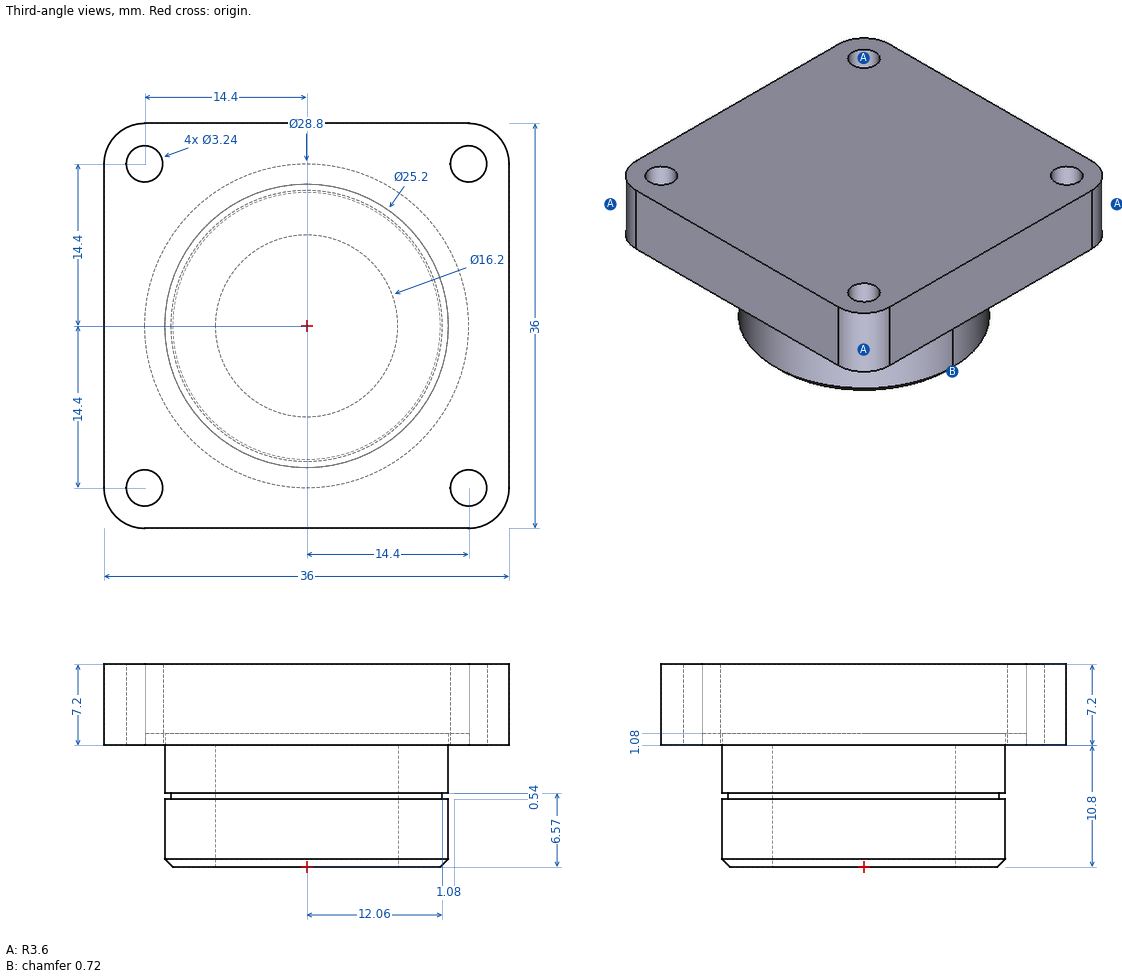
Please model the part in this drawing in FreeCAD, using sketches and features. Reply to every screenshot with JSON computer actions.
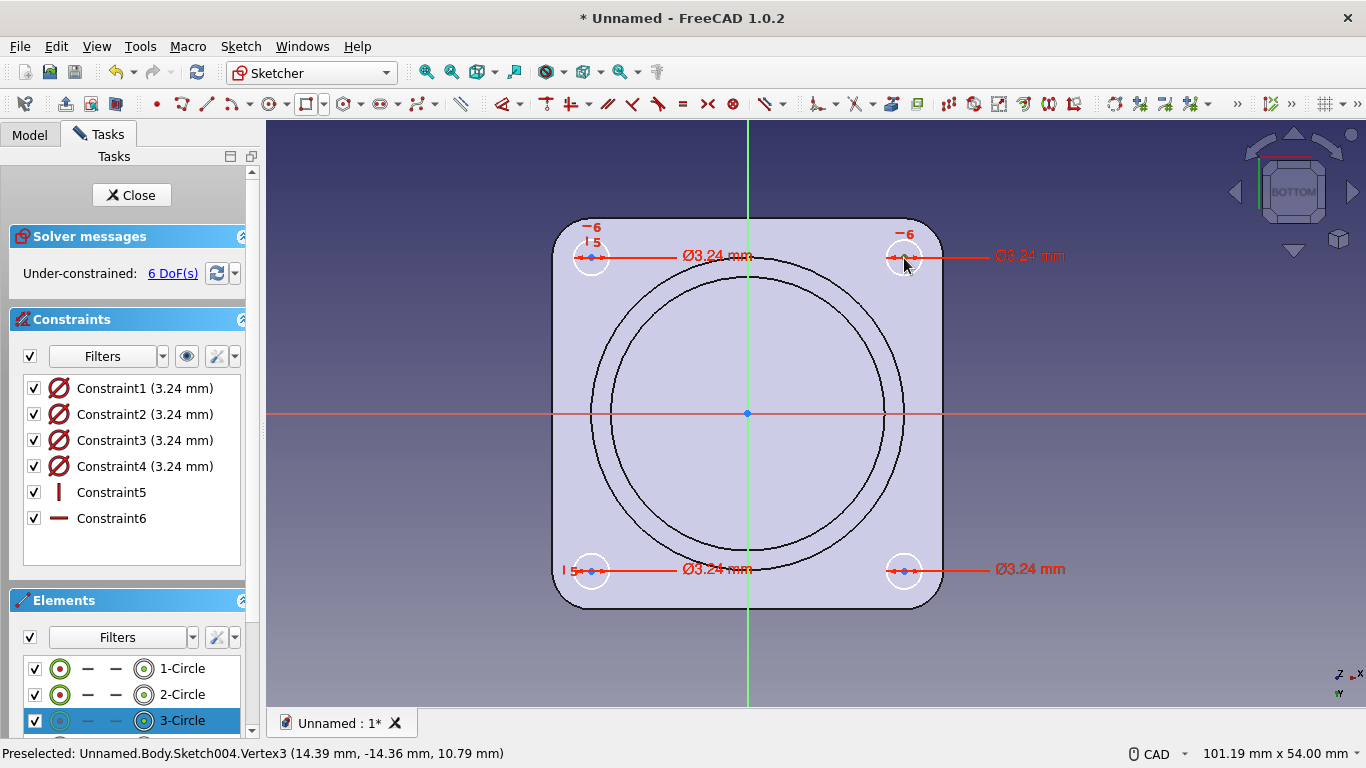
{"action": "left_click", "coordinate": [904, 571]}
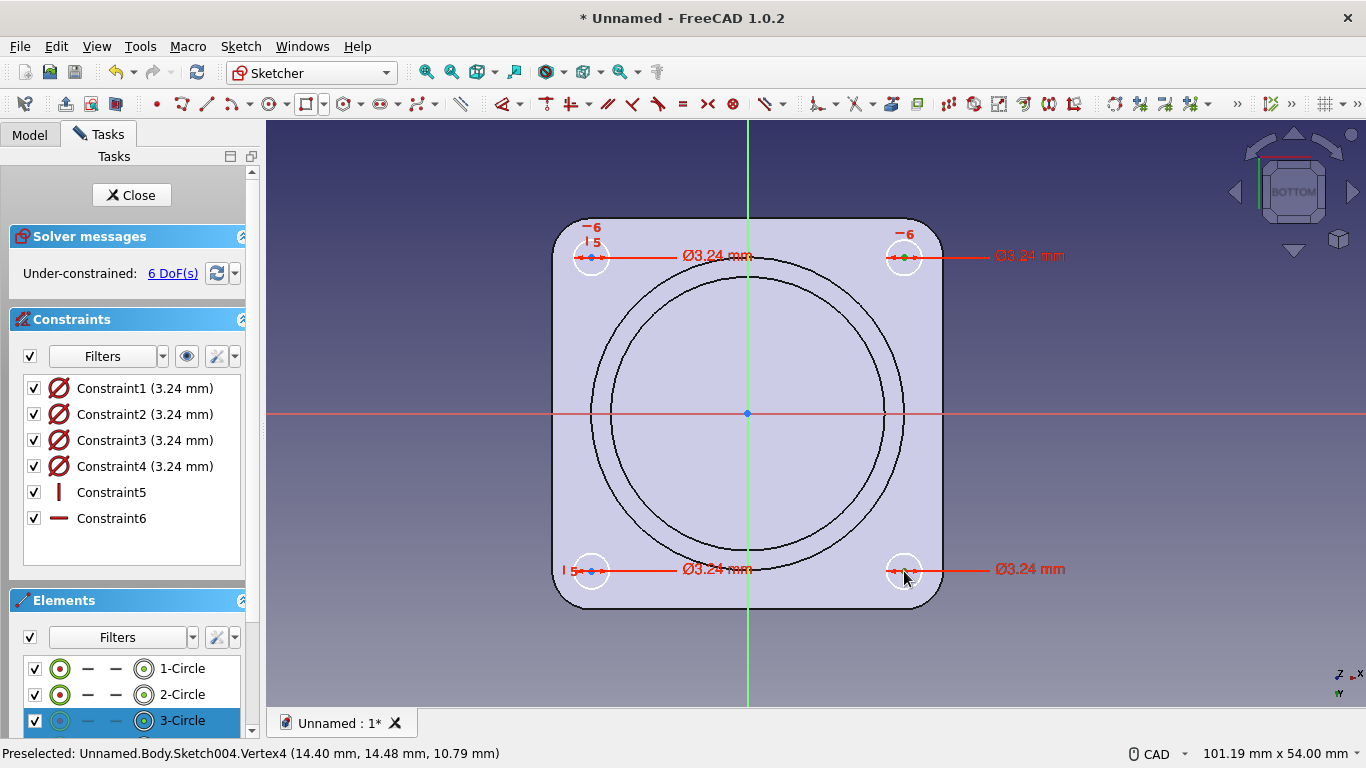
{"action": "left_click", "coordinate": [588, 104]}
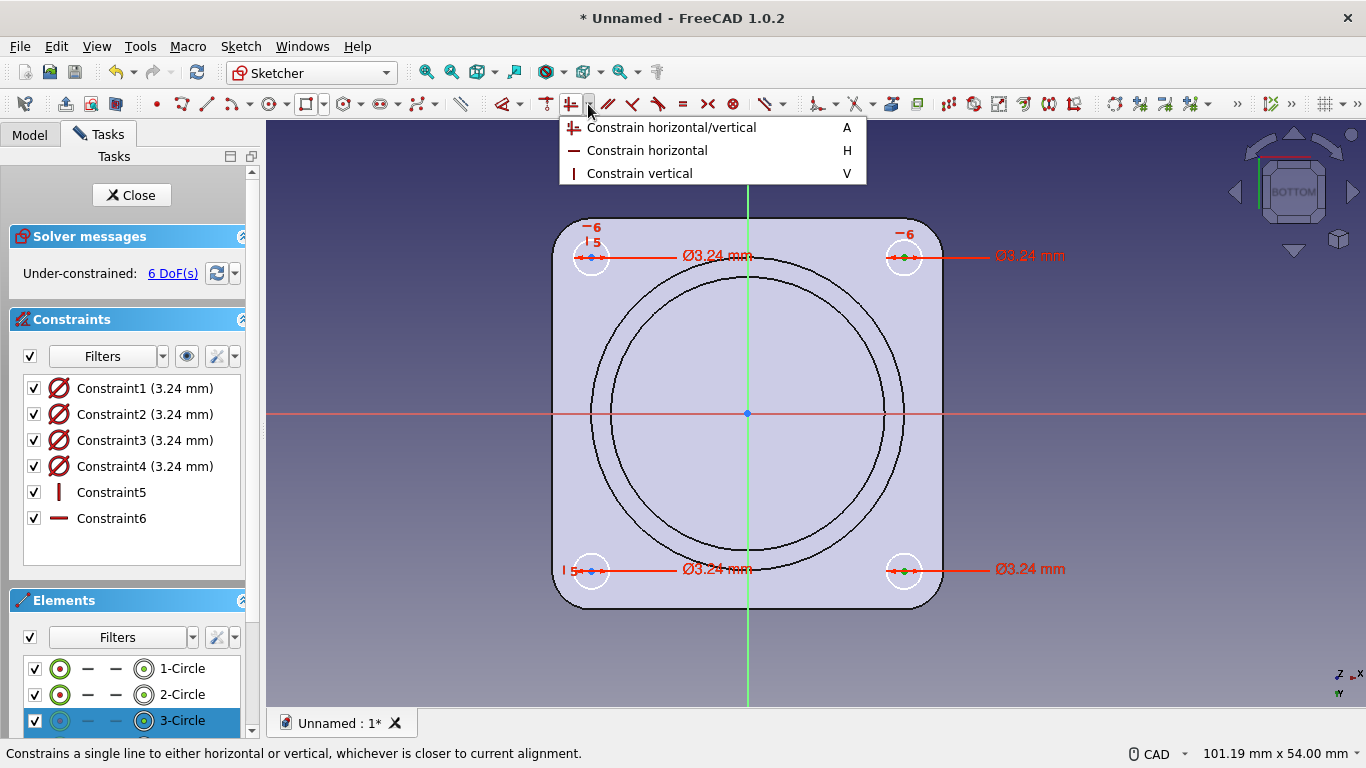
{"action": "left_click", "coordinate": [713, 174]}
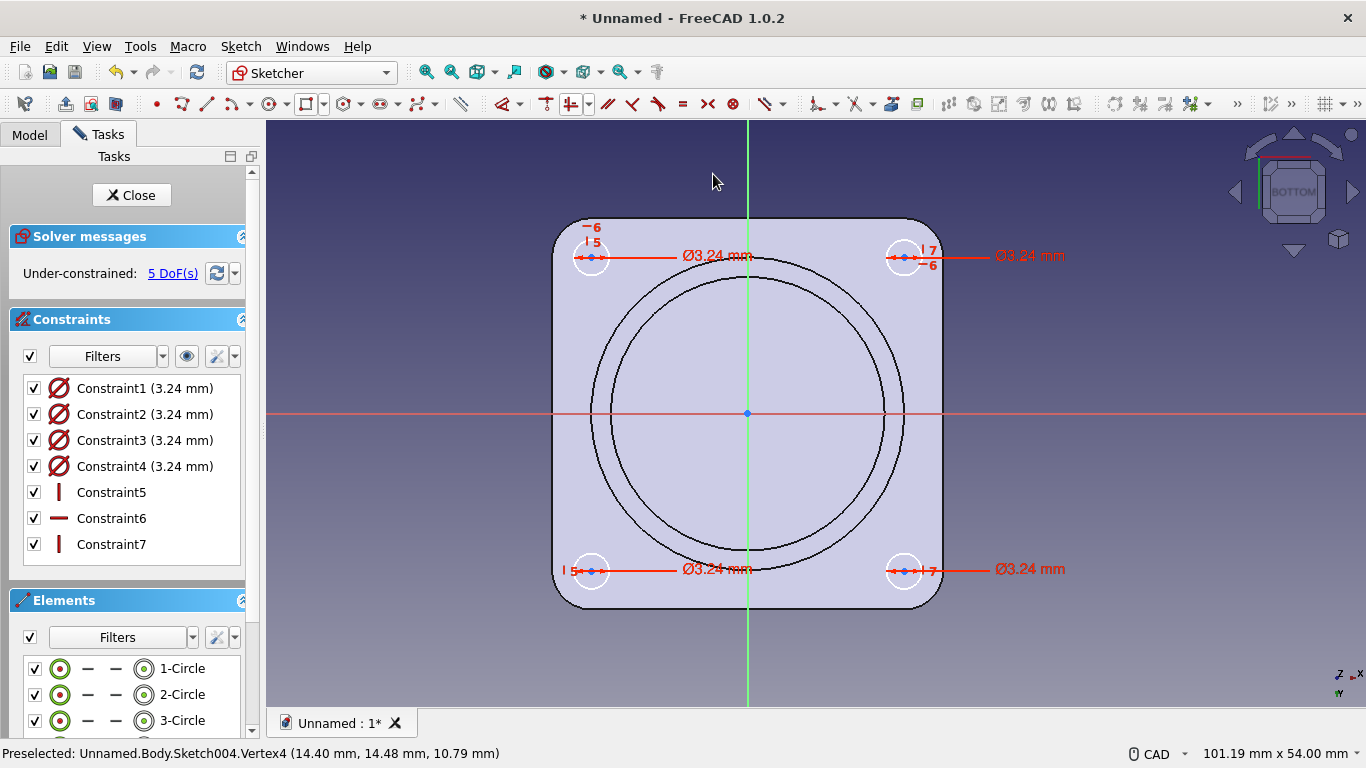
{"action": "left_click", "coordinate": [591, 571]}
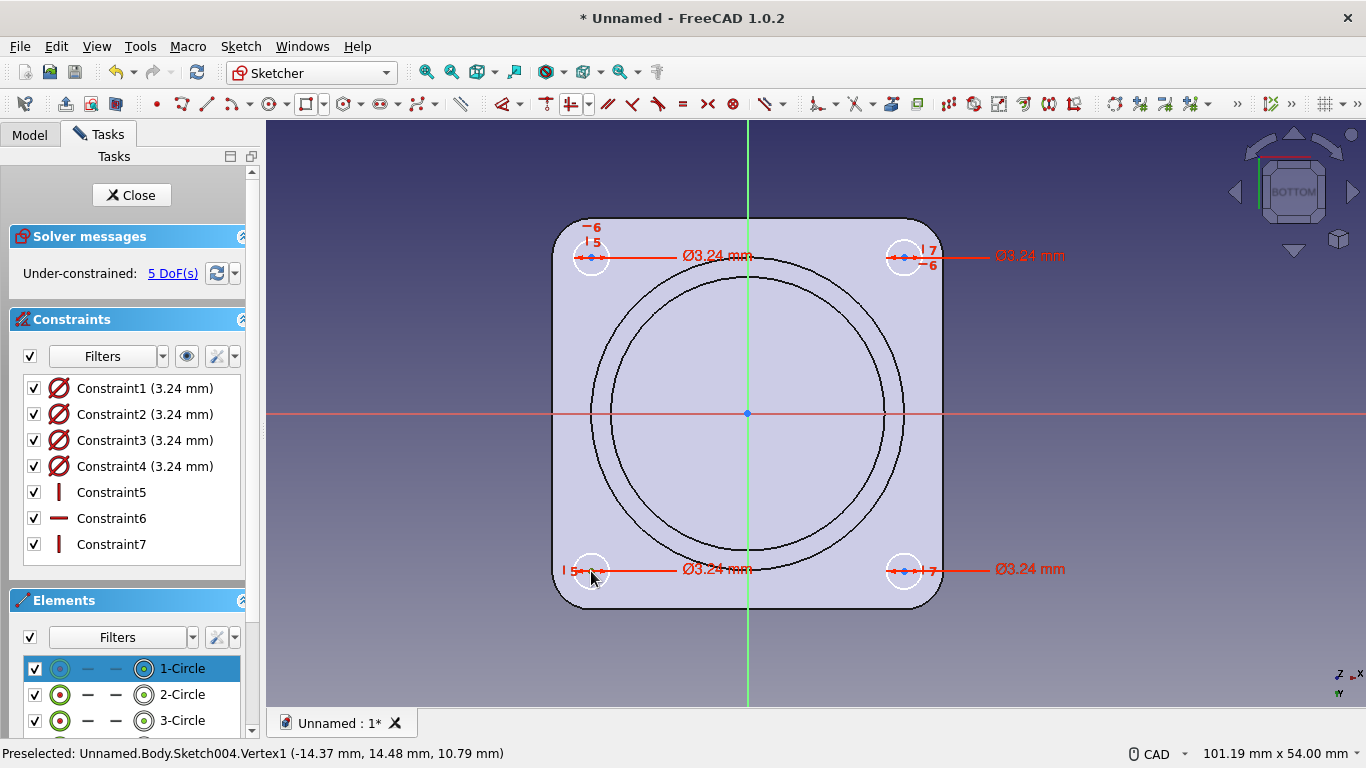
{"action": "left_click", "coordinate": [904, 571]}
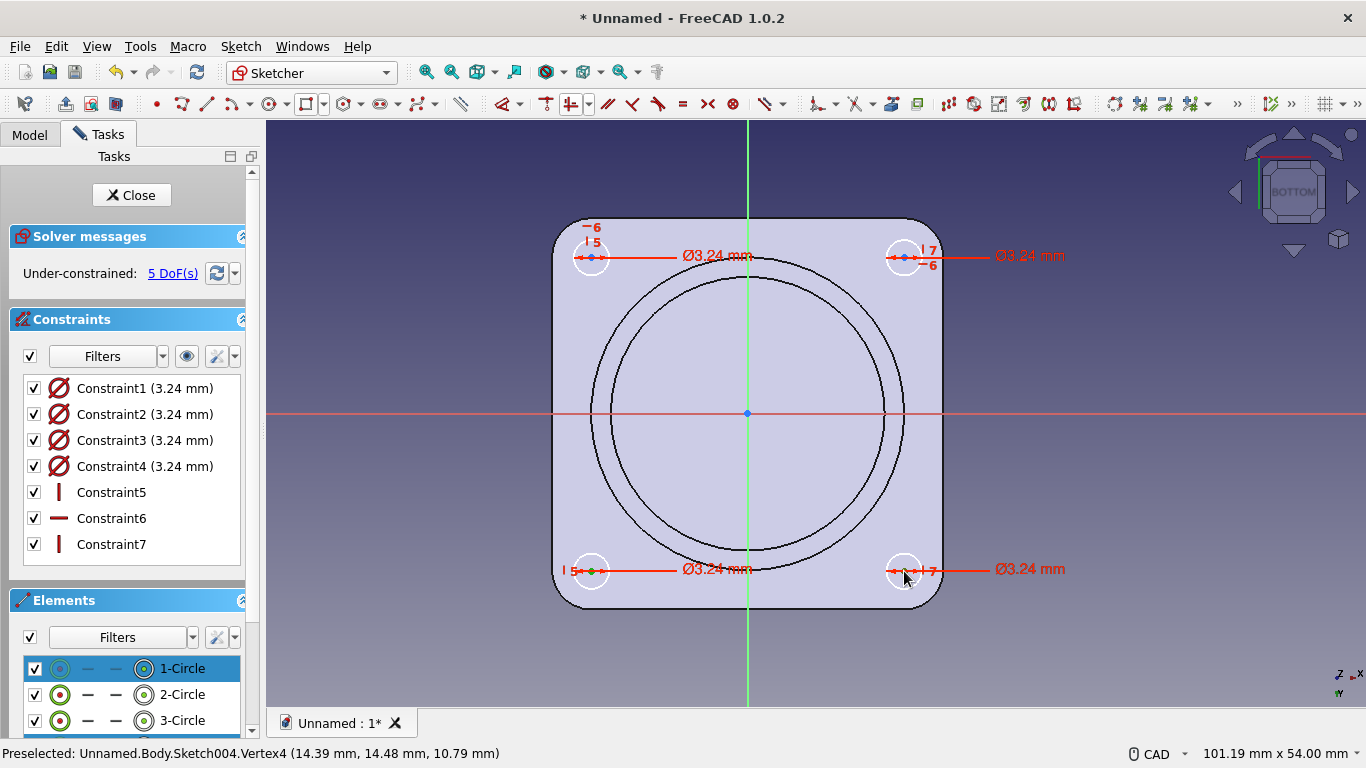
{"action": "left_click", "coordinate": [588, 104]}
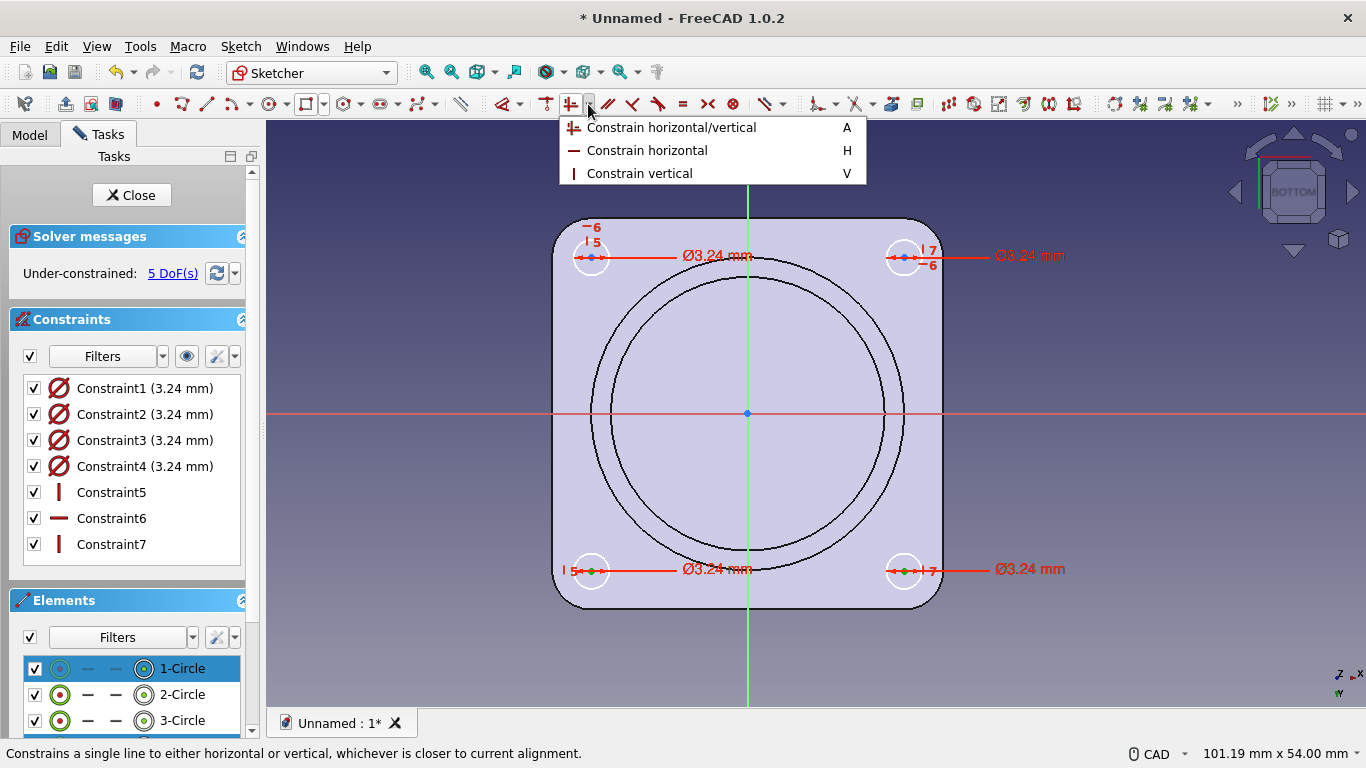
{"action": "left_click", "coordinate": [713, 150]}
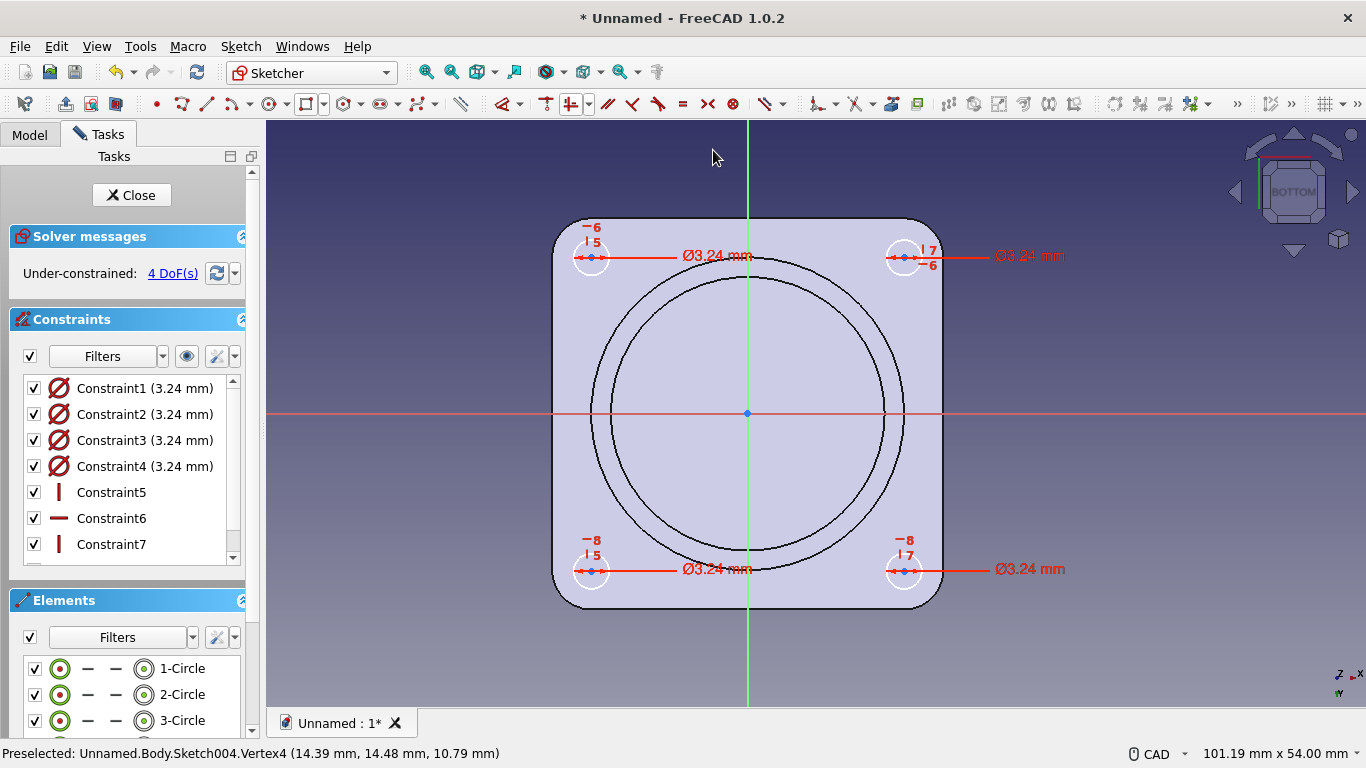
{"action": "key", "text": "d"}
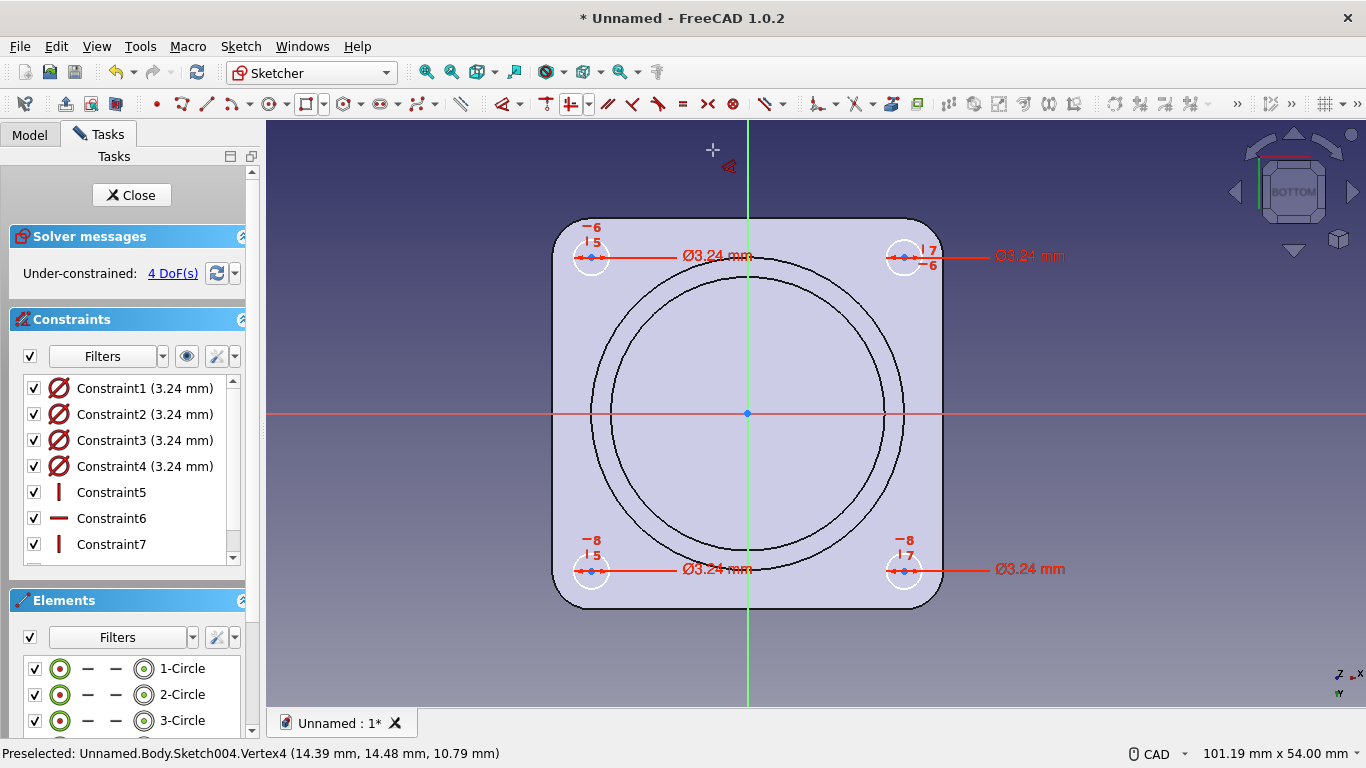
{"action": "left_click", "coordinate": [591, 571]}
{"action": "left_click", "coordinate": [670, 605]}